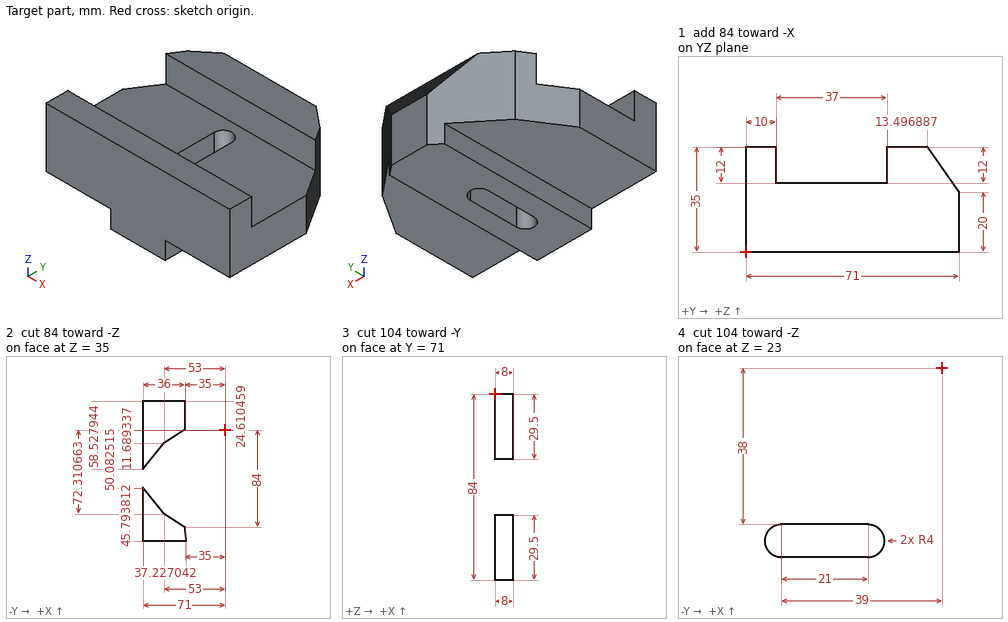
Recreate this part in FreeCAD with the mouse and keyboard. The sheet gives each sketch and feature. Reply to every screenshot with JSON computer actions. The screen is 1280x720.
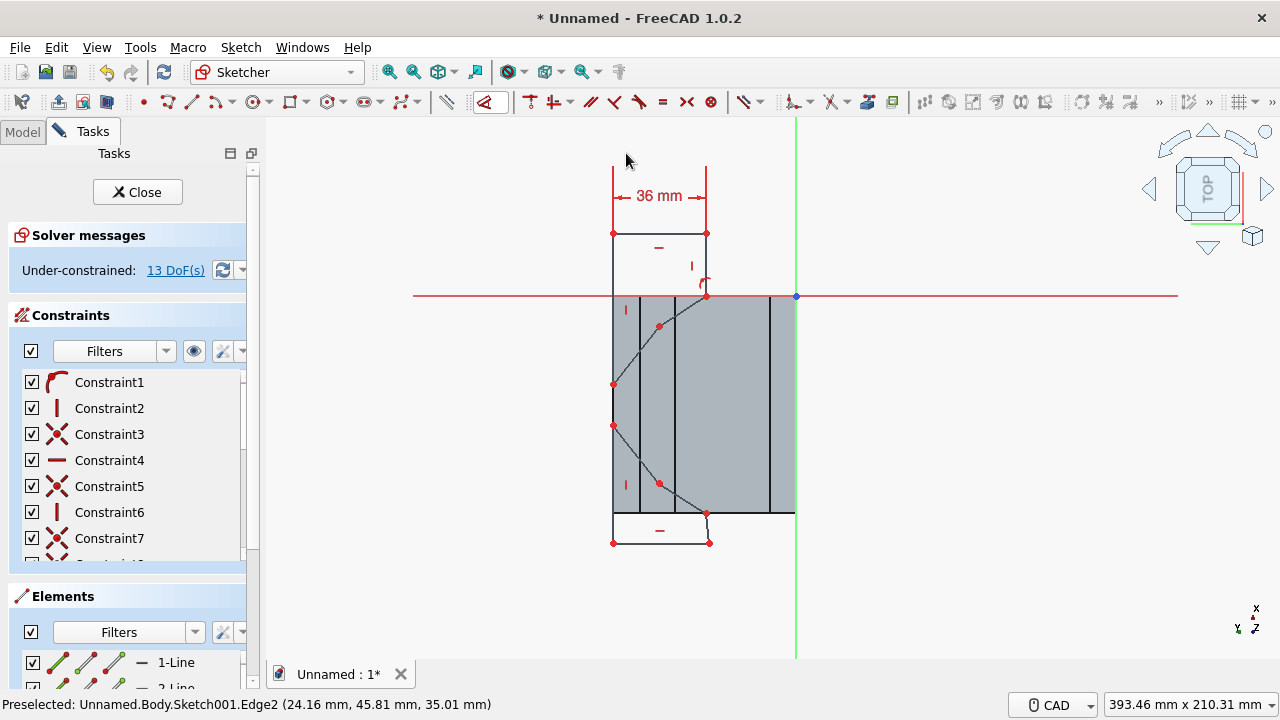
{"action": "left_click", "coordinate": [706, 296]}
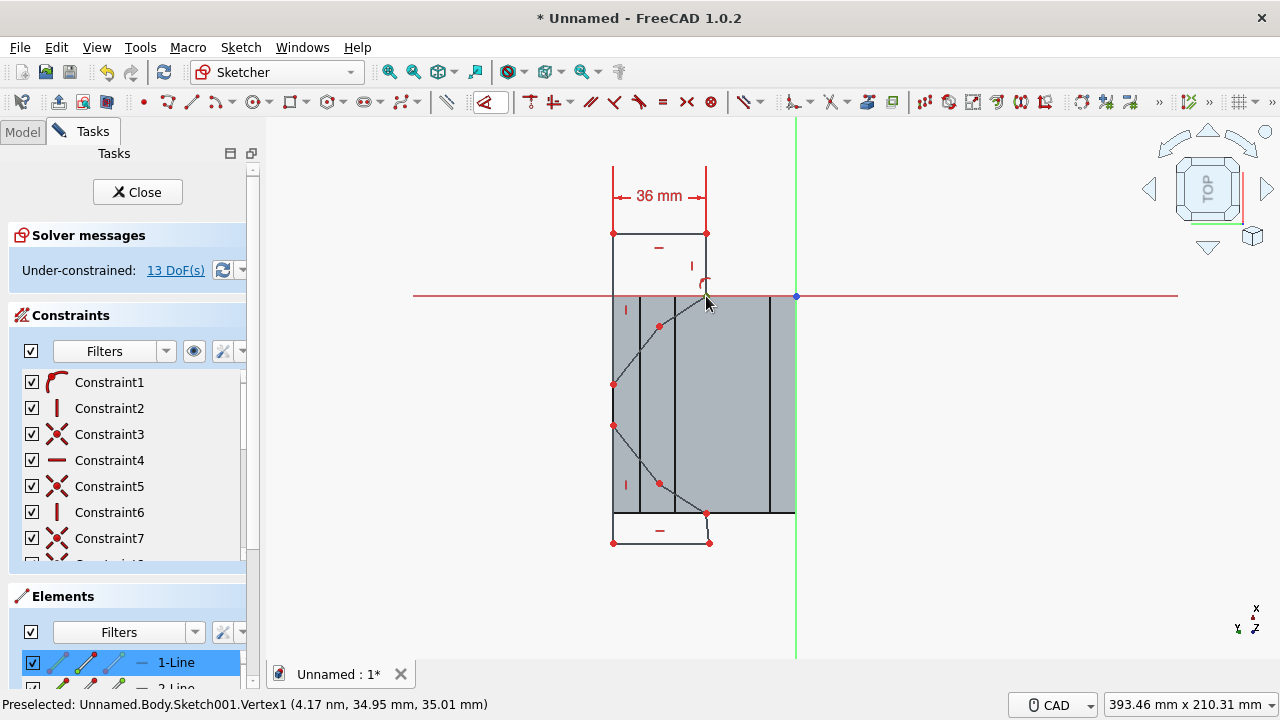
{"action": "left_click", "coordinate": [502, 102]}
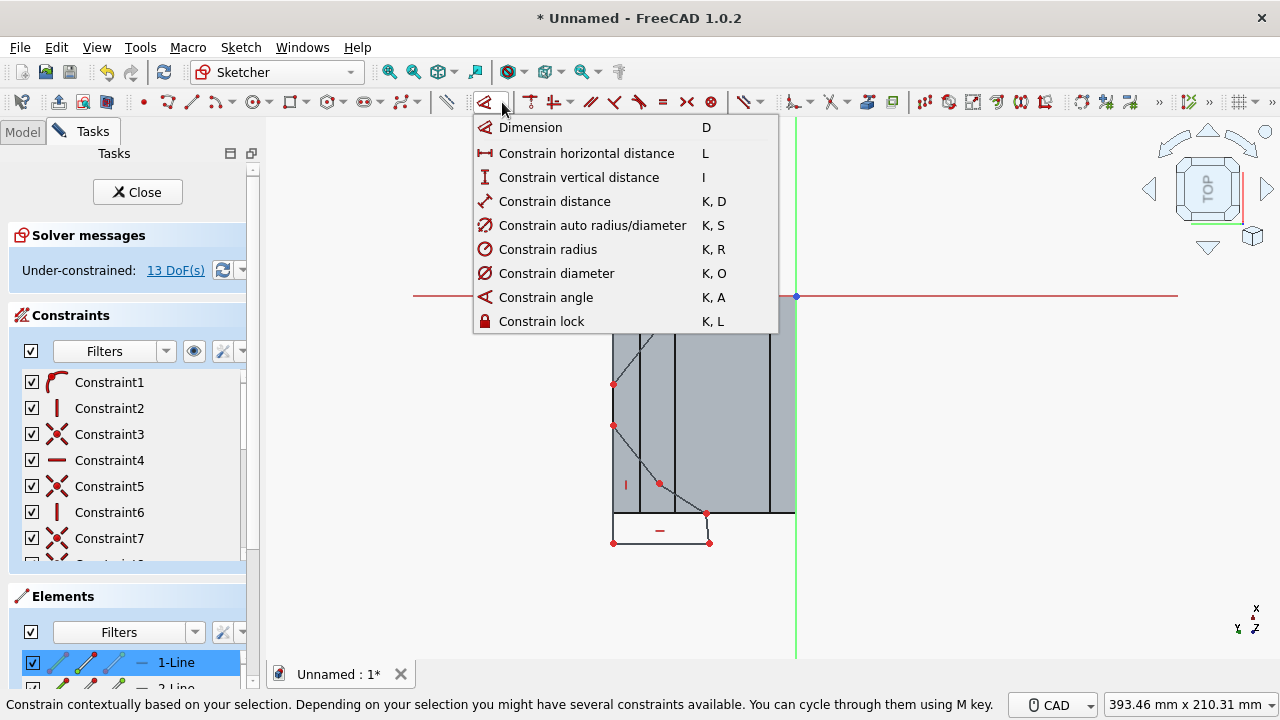
{"action": "left_click", "coordinate": [626, 153]}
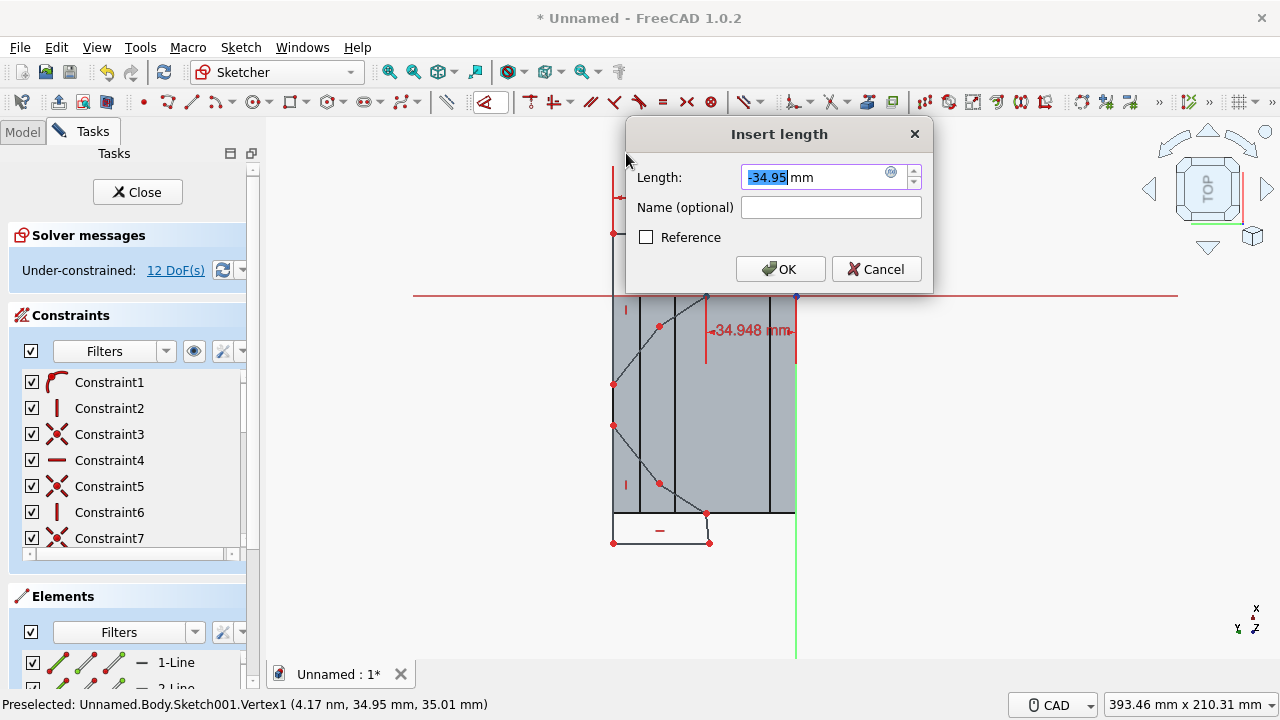
{"action": "type", "text": "-35"}
{"action": "key", "text": "Return"}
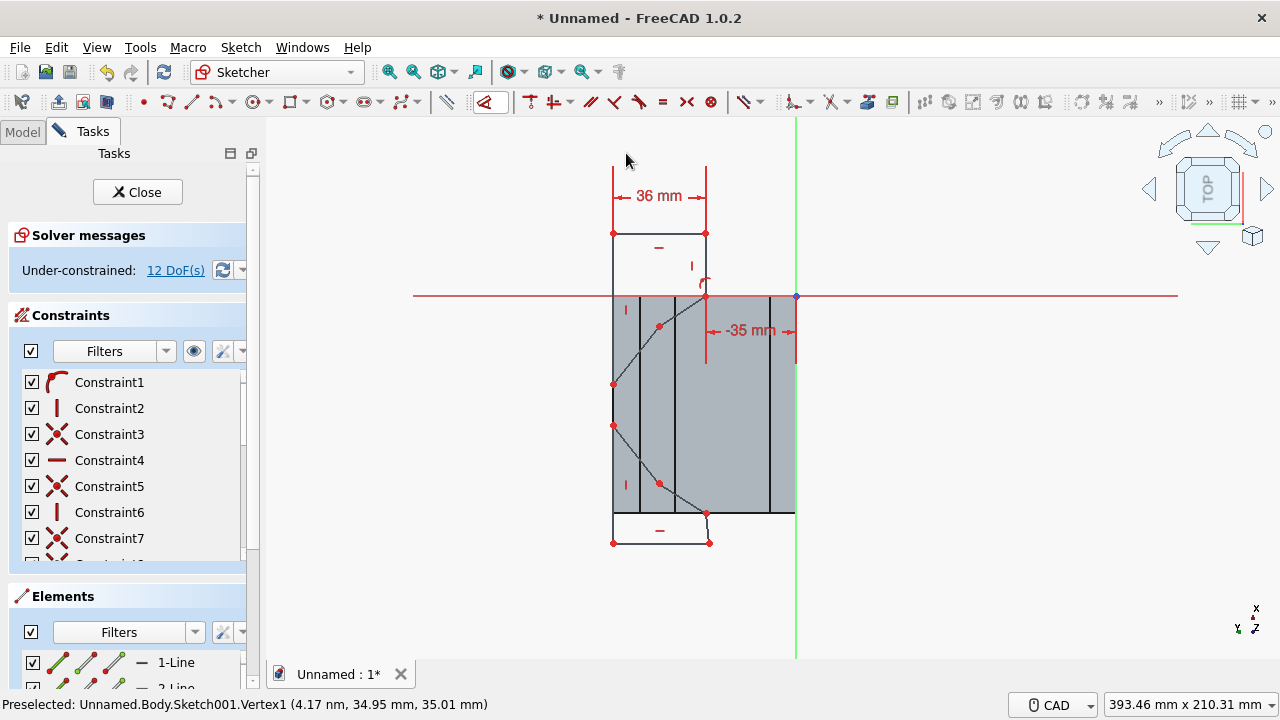
{"action": "left_click", "coordinate": [659, 327]}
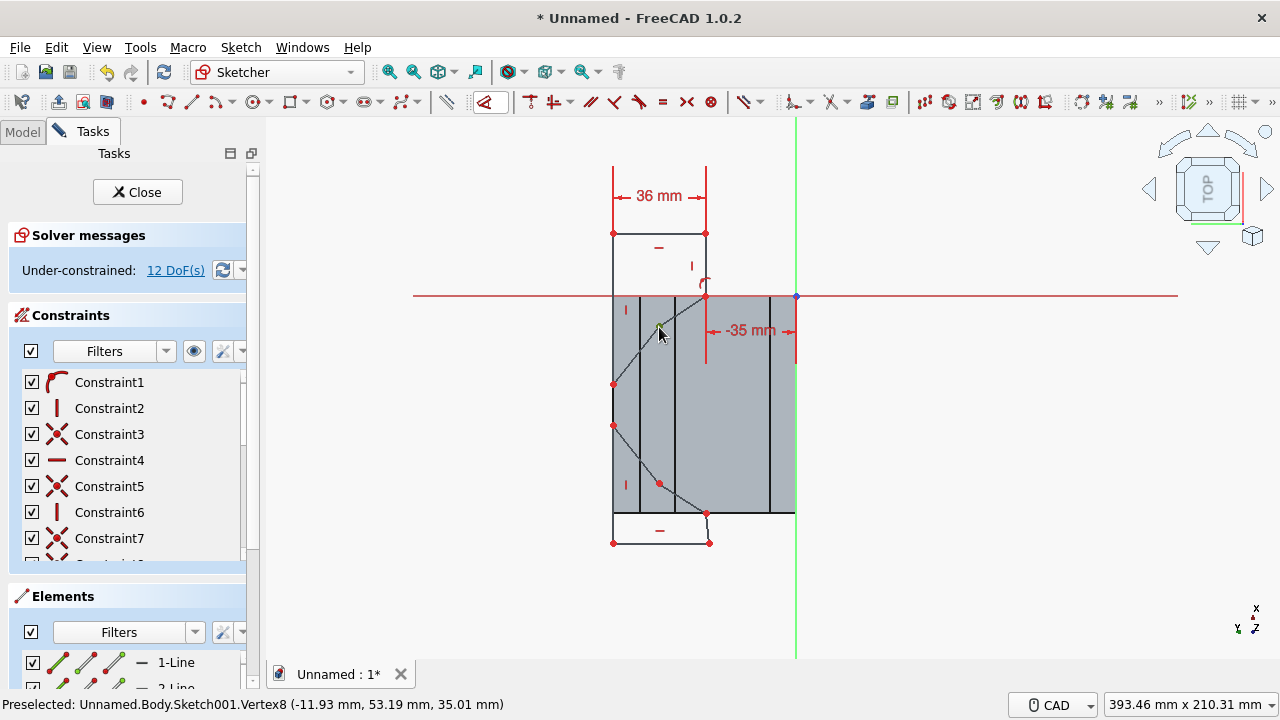
{"action": "left_click", "coordinate": [502, 102]}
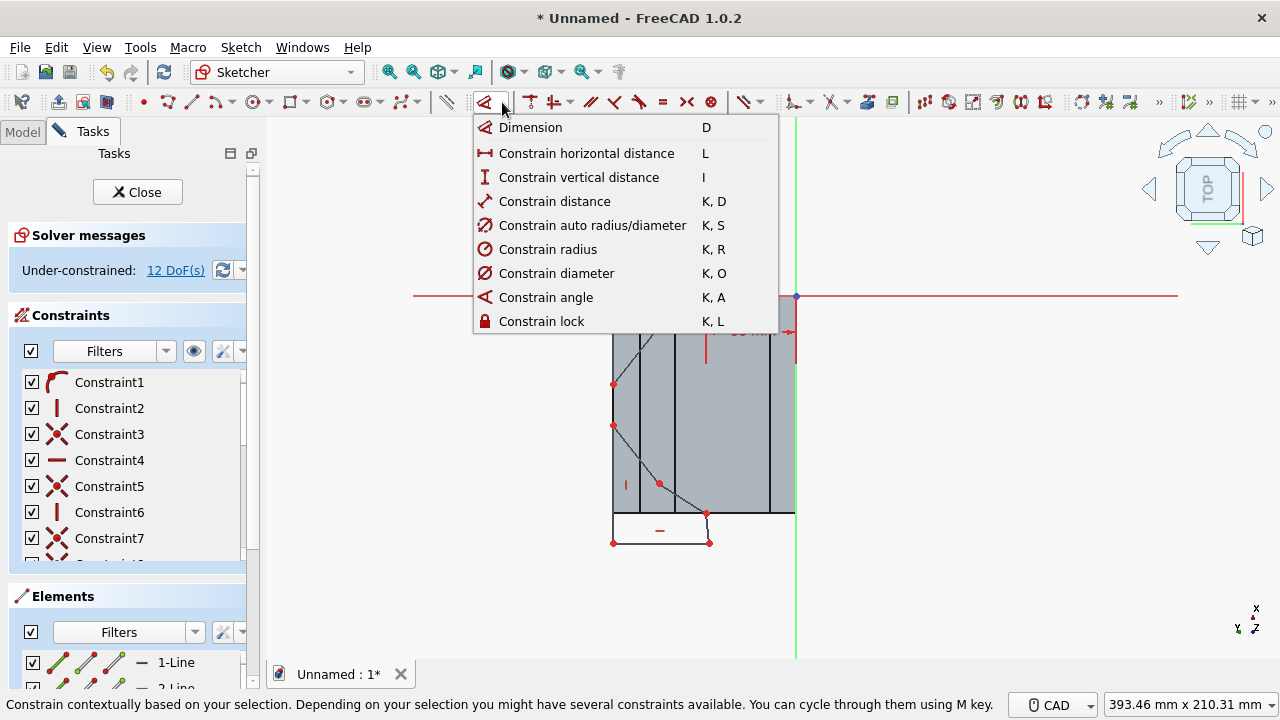
{"action": "left_click", "coordinate": [626, 153]}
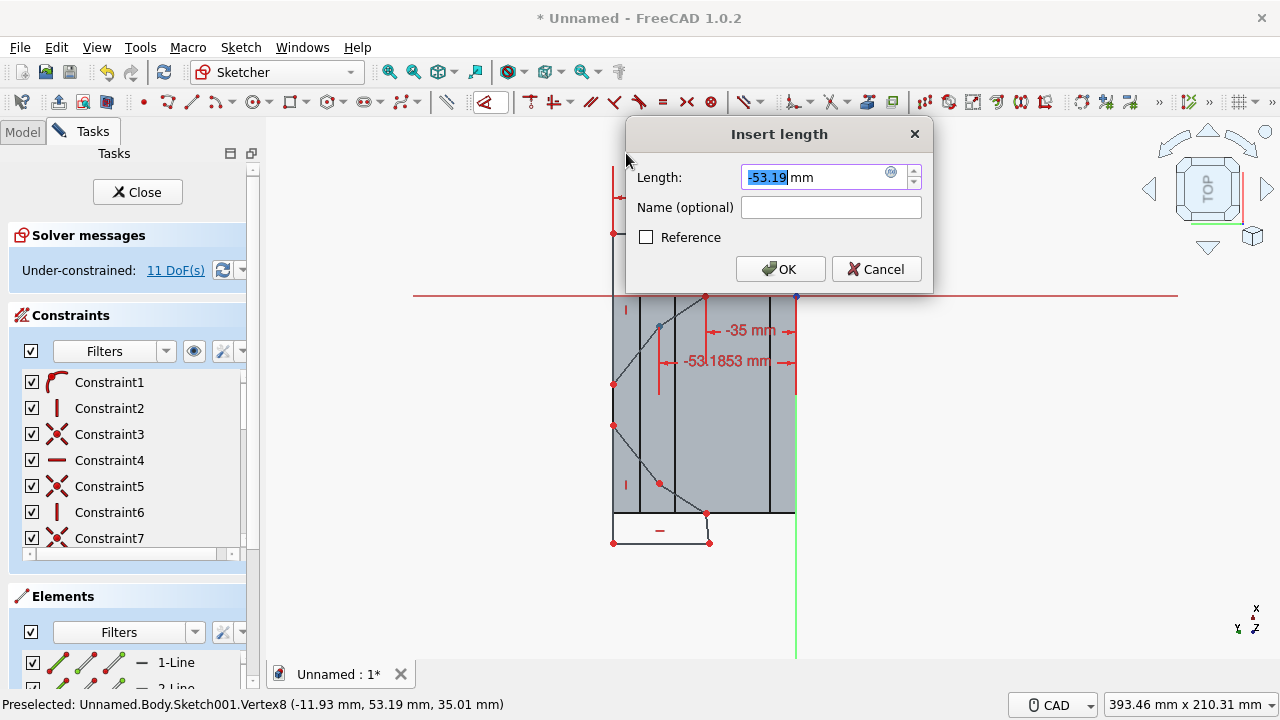
{"action": "type", "text": "-53"}
{"action": "key", "text": "Return"}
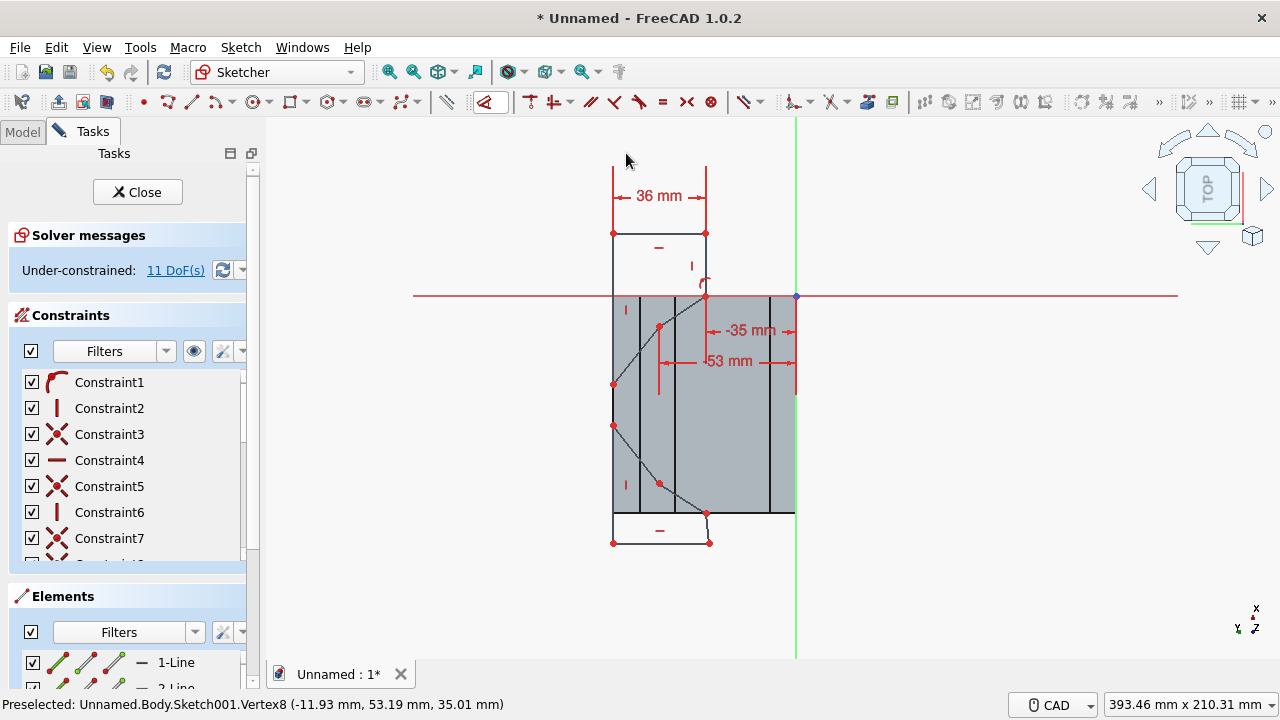
{"action": "left_click", "coordinate": [613, 426]}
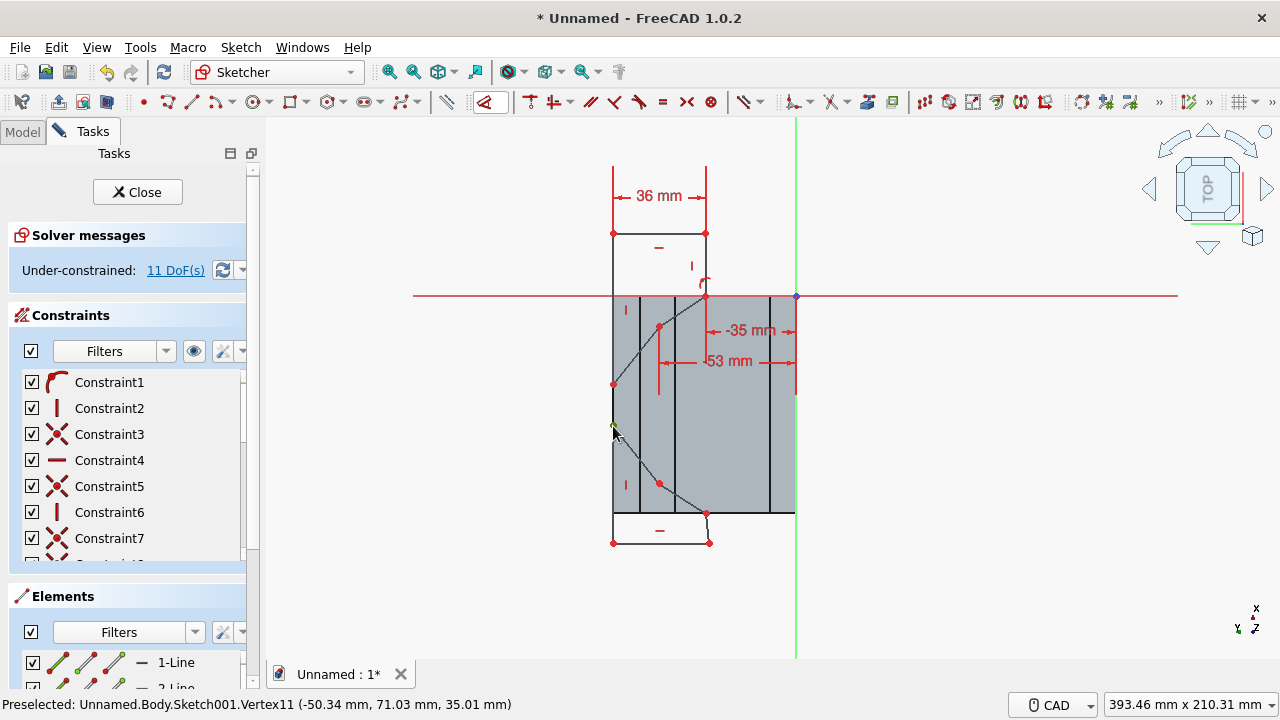
{"action": "left_click", "coordinate": [502, 102]}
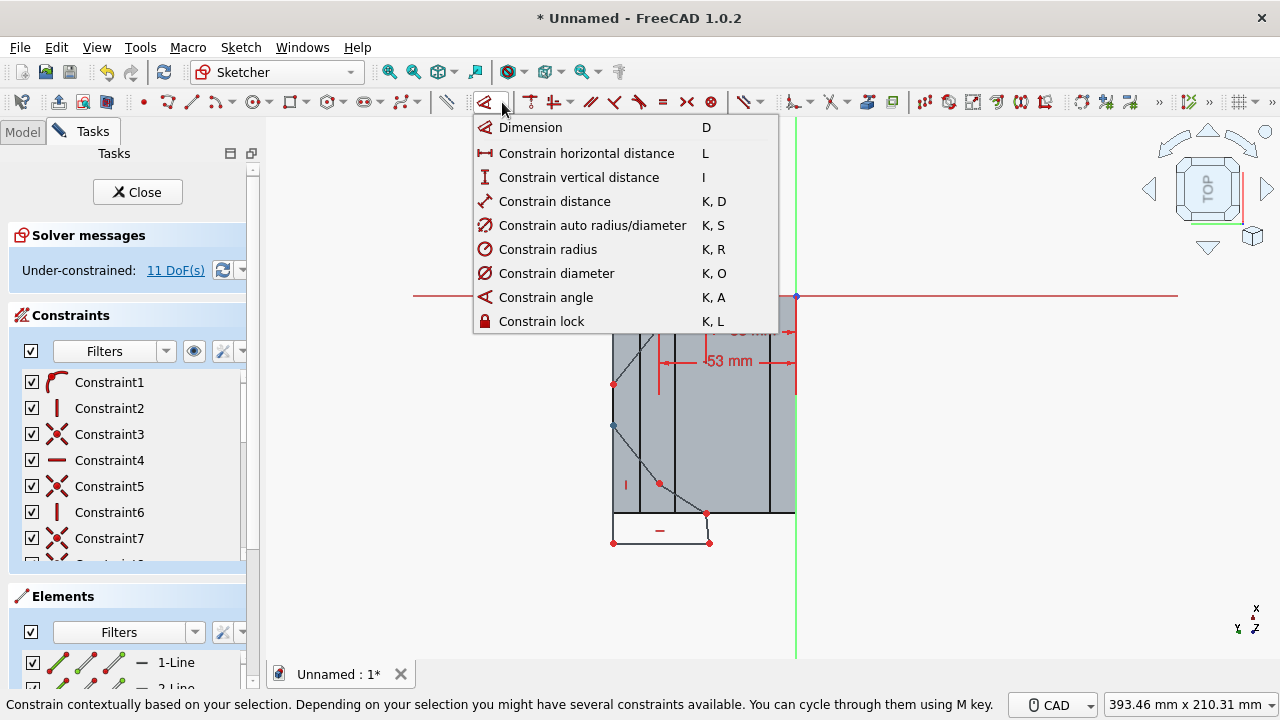
{"action": "left_click", "coordinate": [626, 153]}